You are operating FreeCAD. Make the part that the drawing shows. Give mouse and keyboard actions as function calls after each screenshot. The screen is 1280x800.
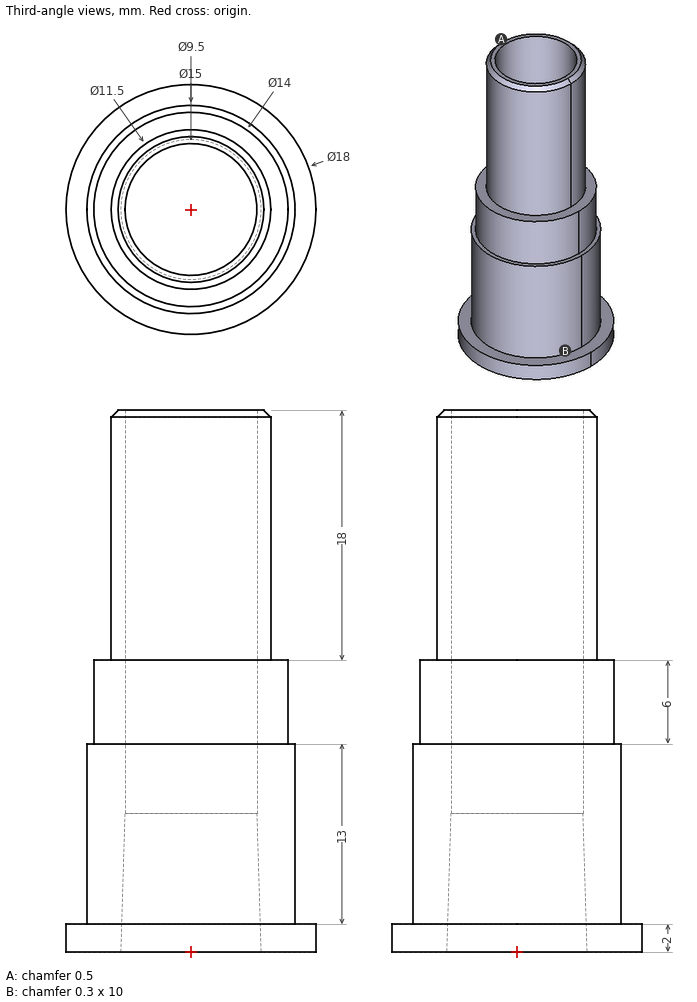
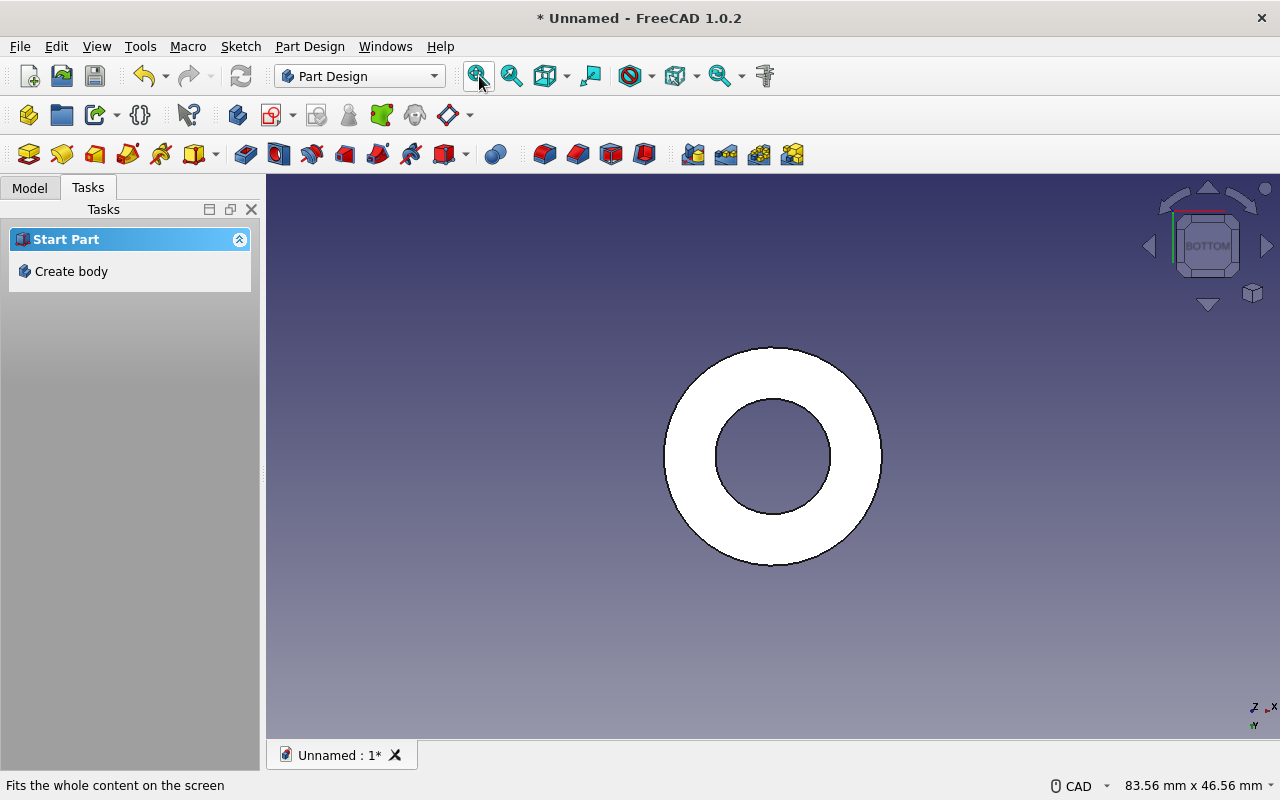
click(715, 455)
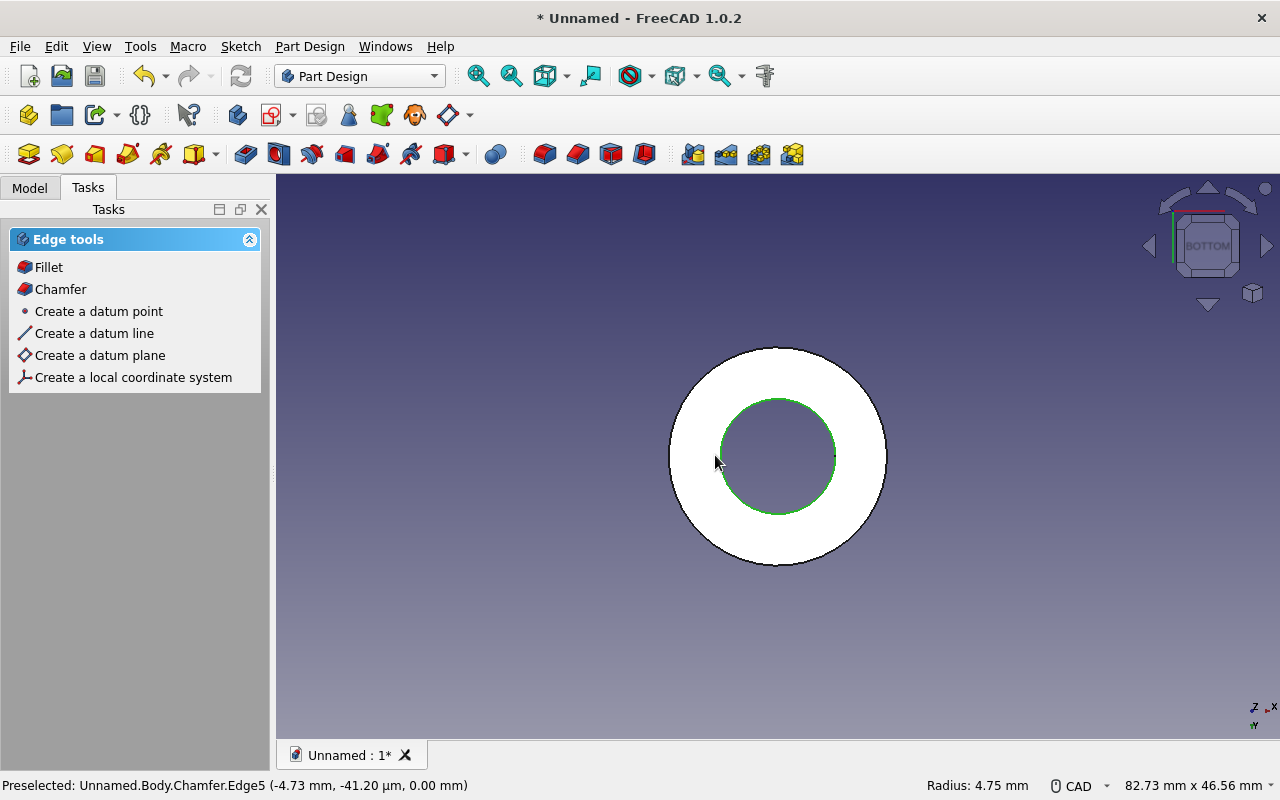
click(578, 154)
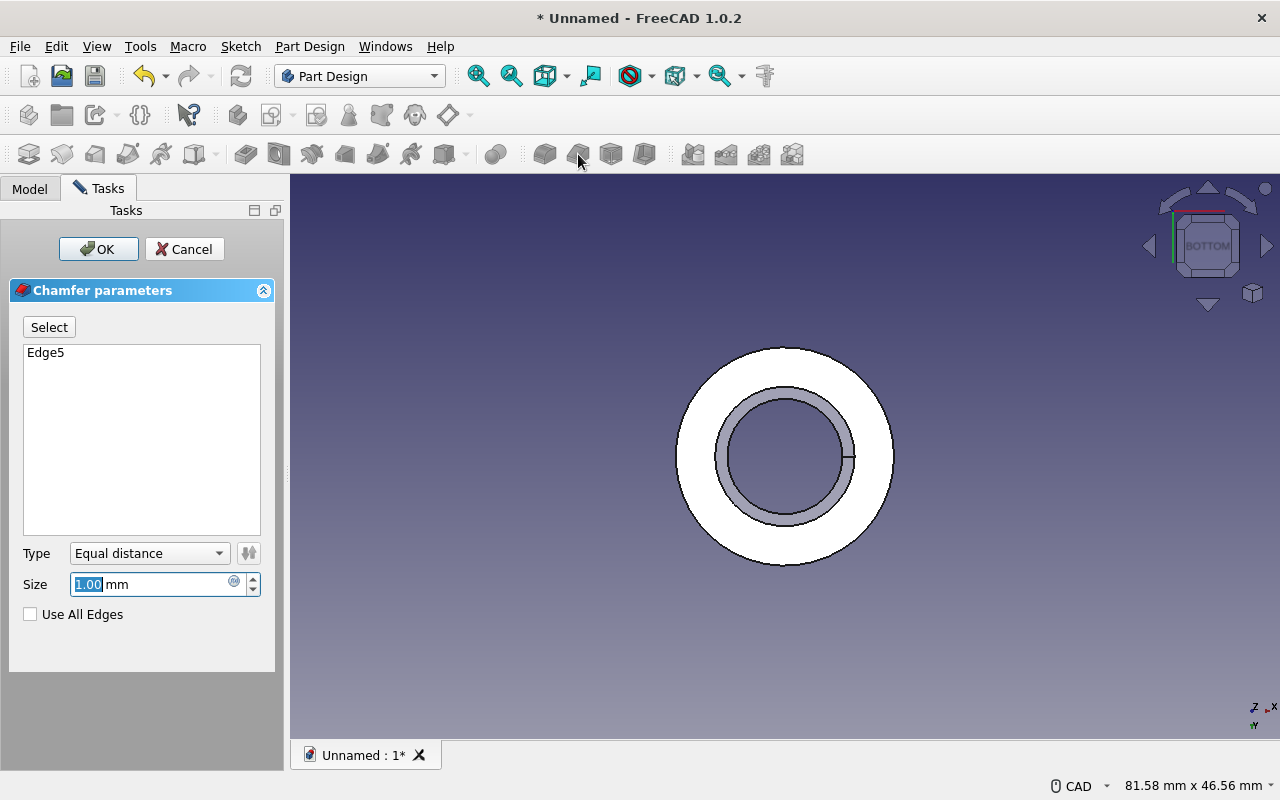
text(0.3)
key(Tab)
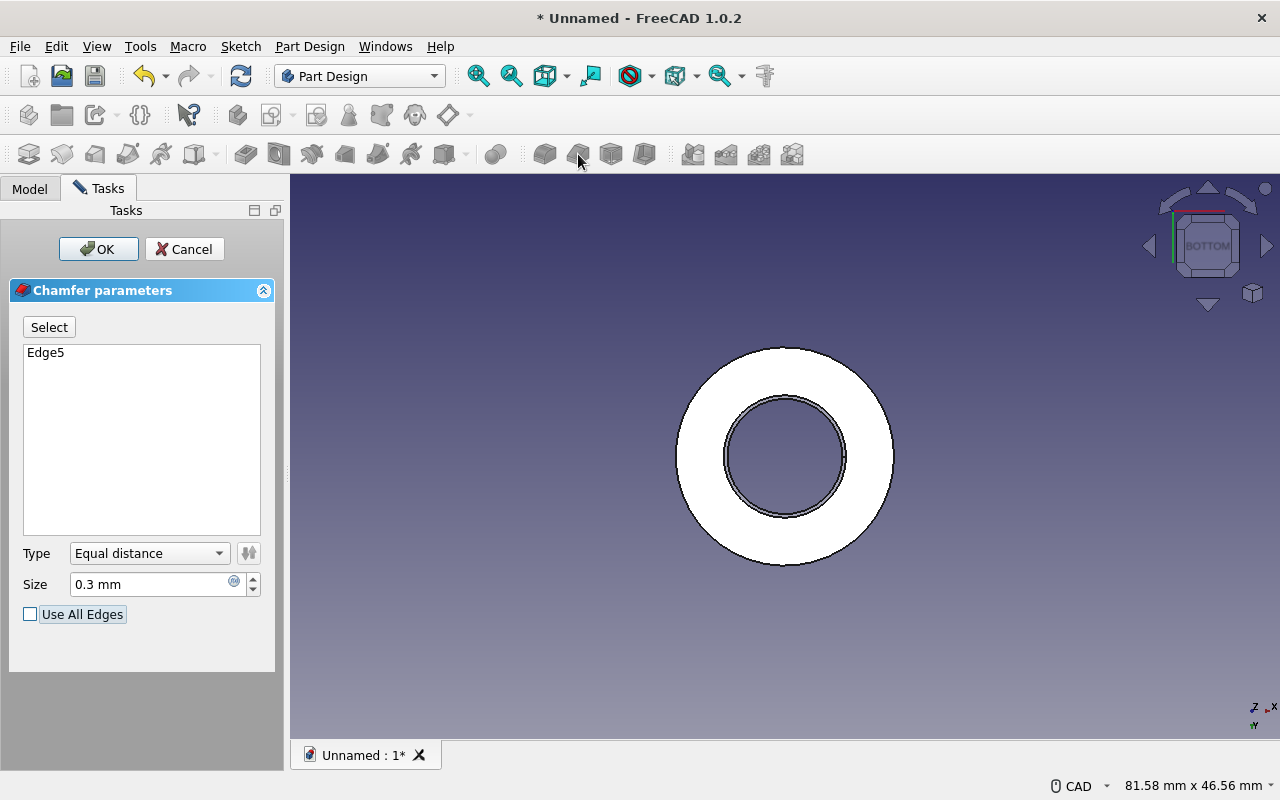
click(150, 554)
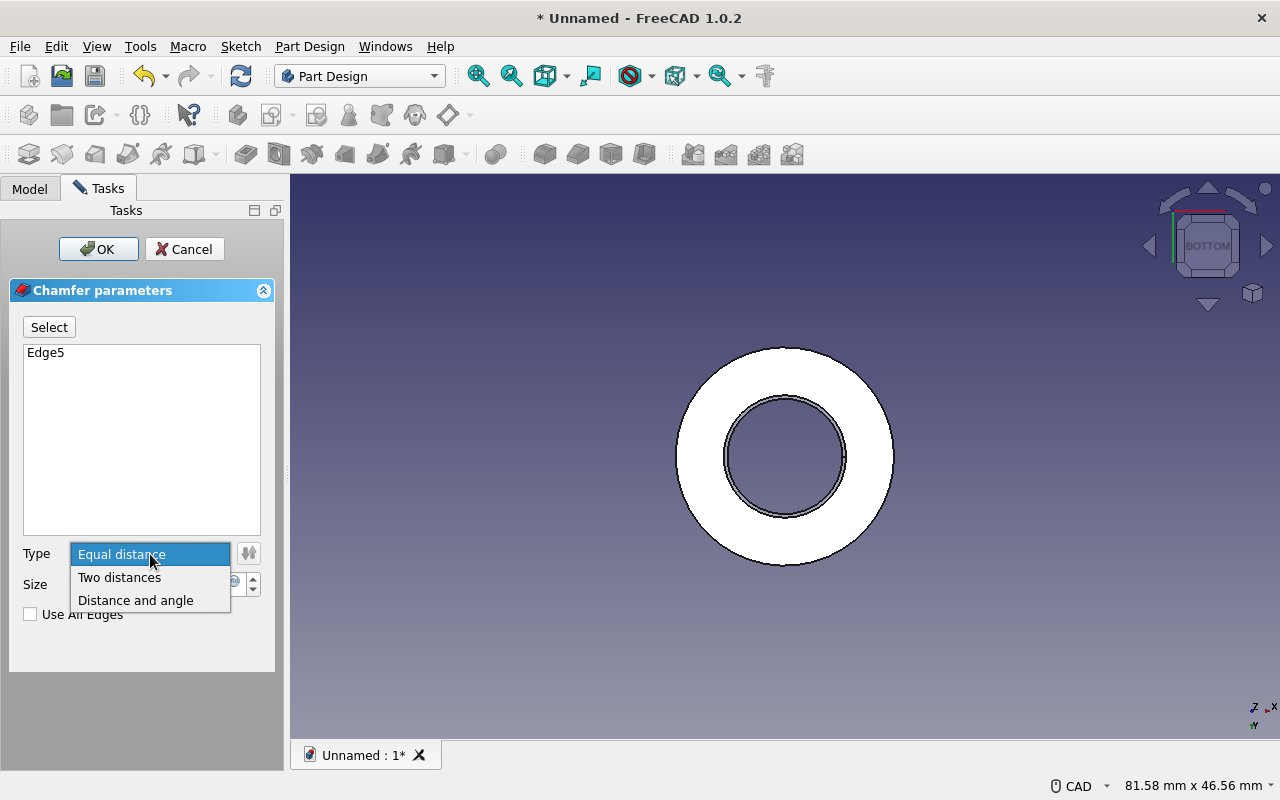
click(148, 578)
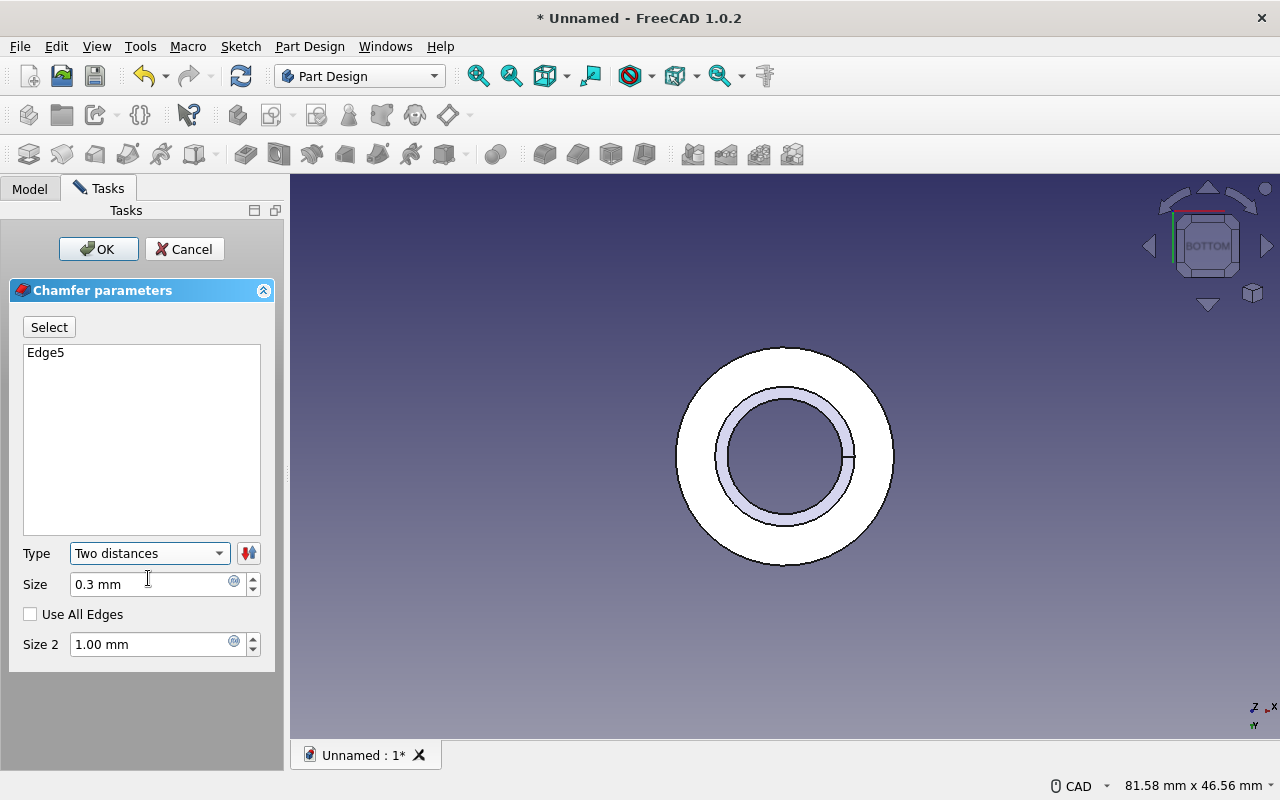
triple_click(158, 644)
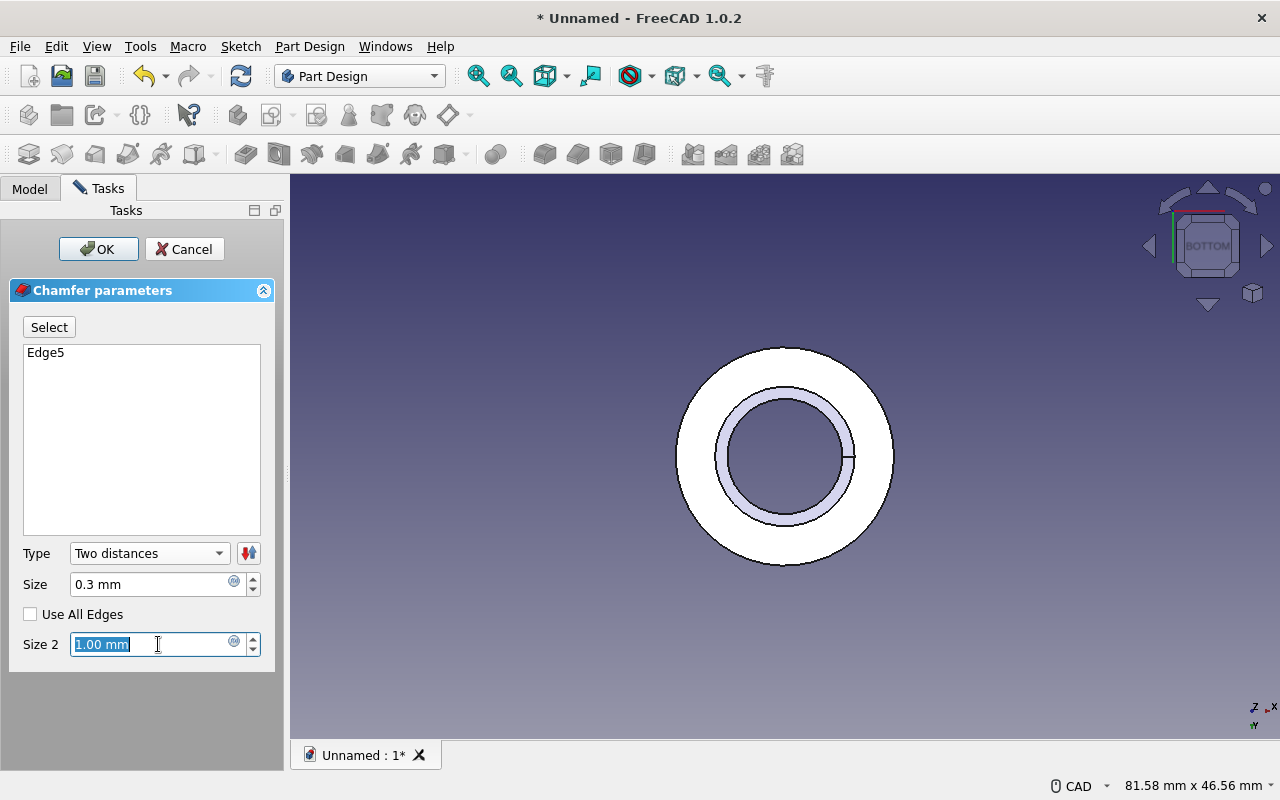
text(10)
key(Tab)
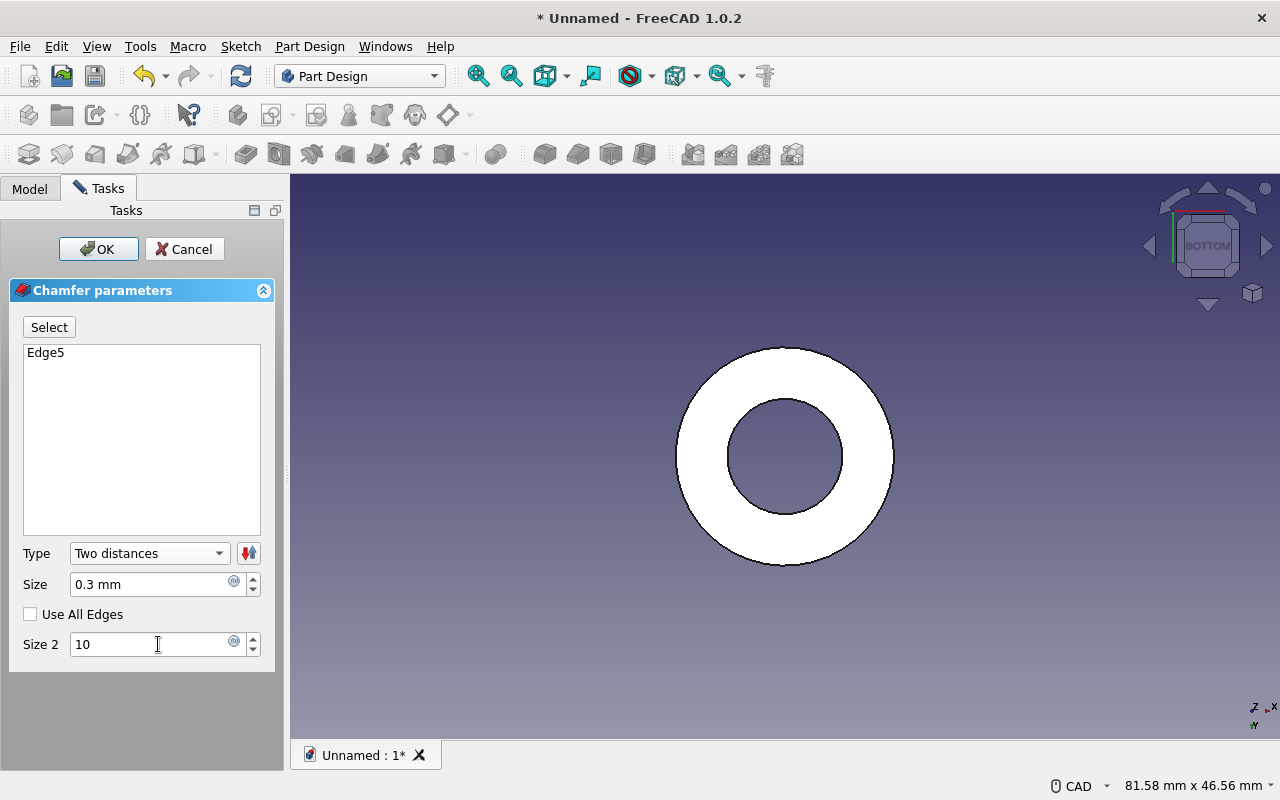
click(249, 554)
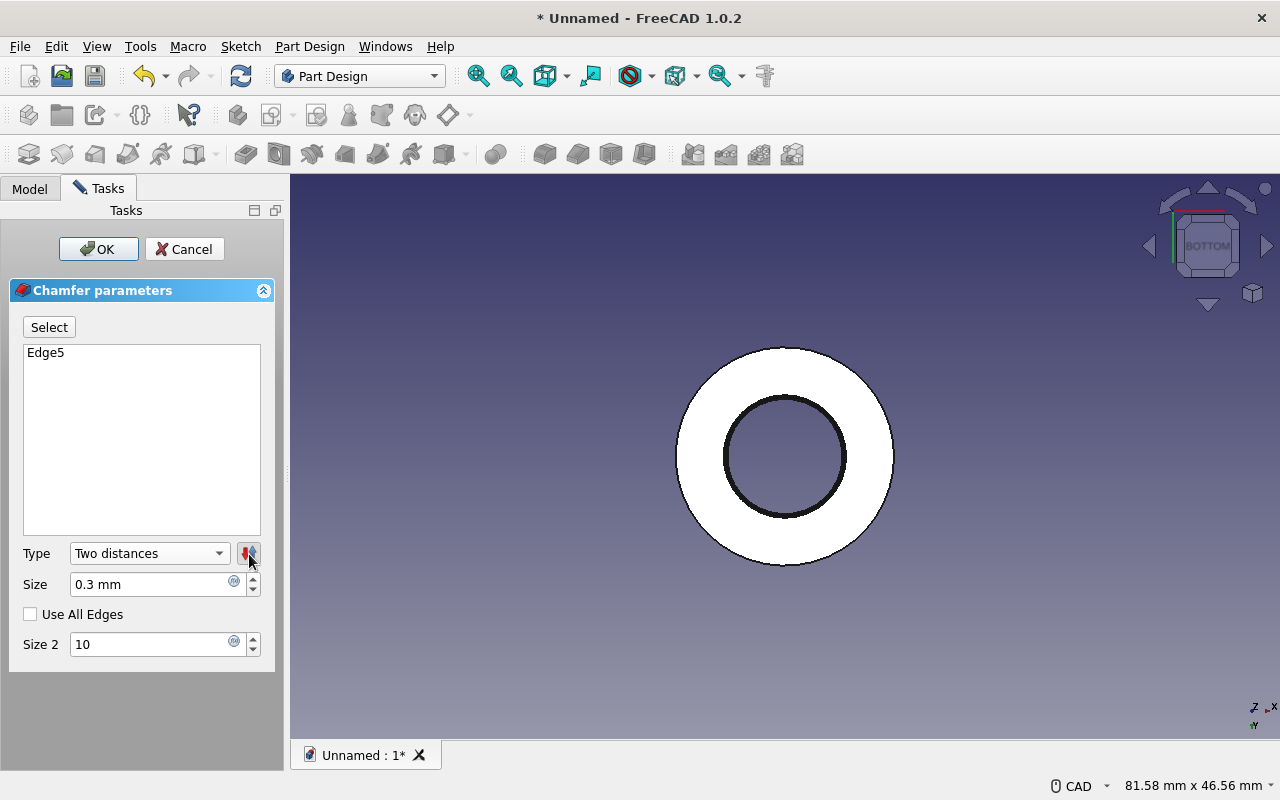
click(99, 249)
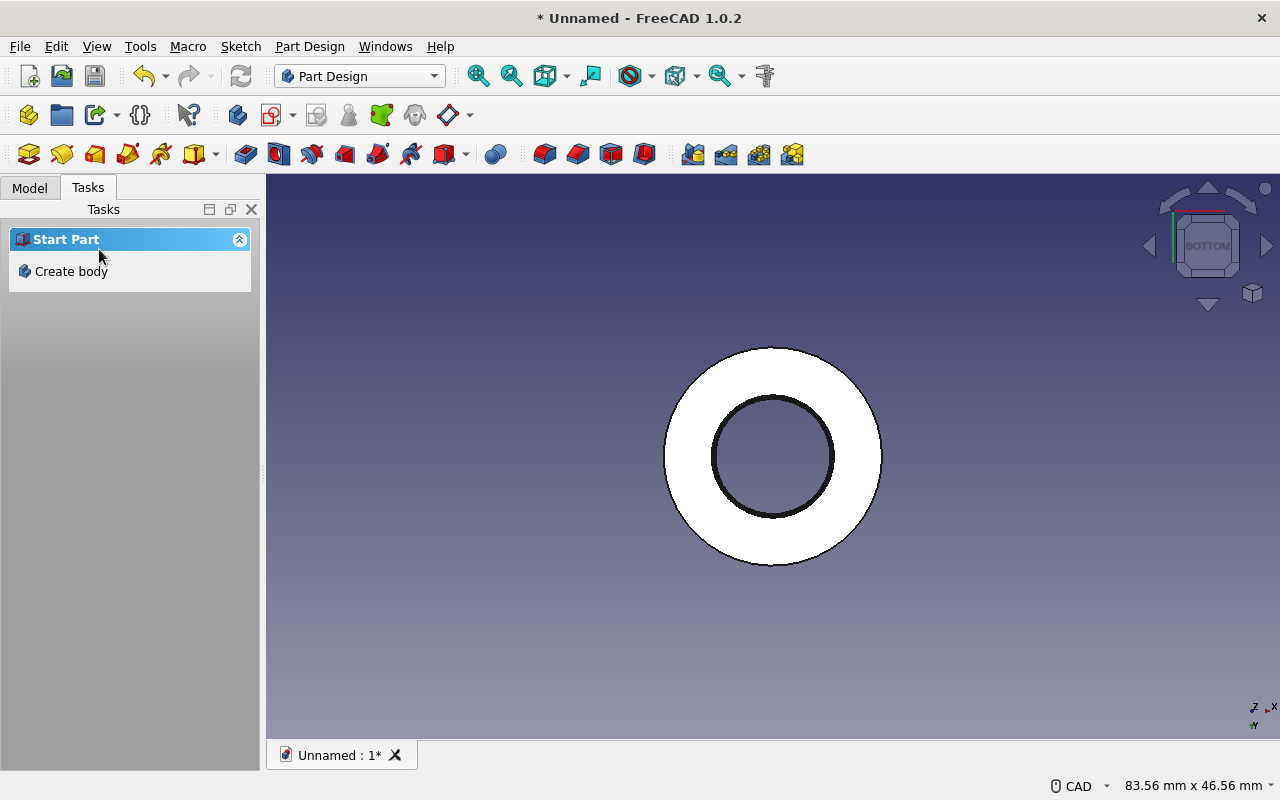
key(0)